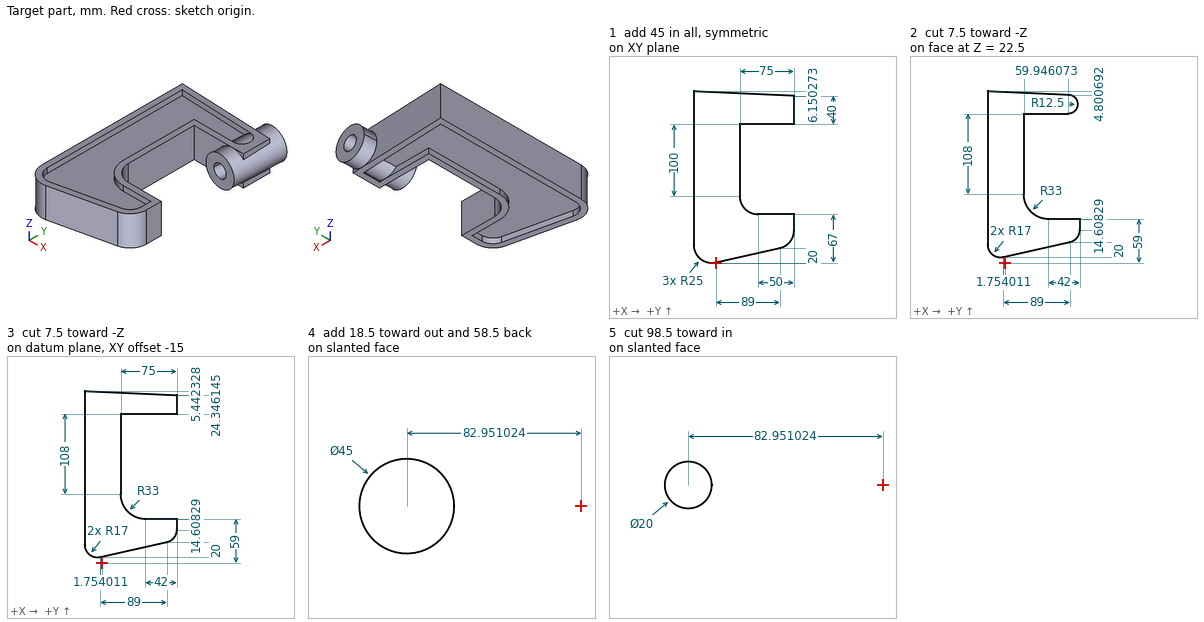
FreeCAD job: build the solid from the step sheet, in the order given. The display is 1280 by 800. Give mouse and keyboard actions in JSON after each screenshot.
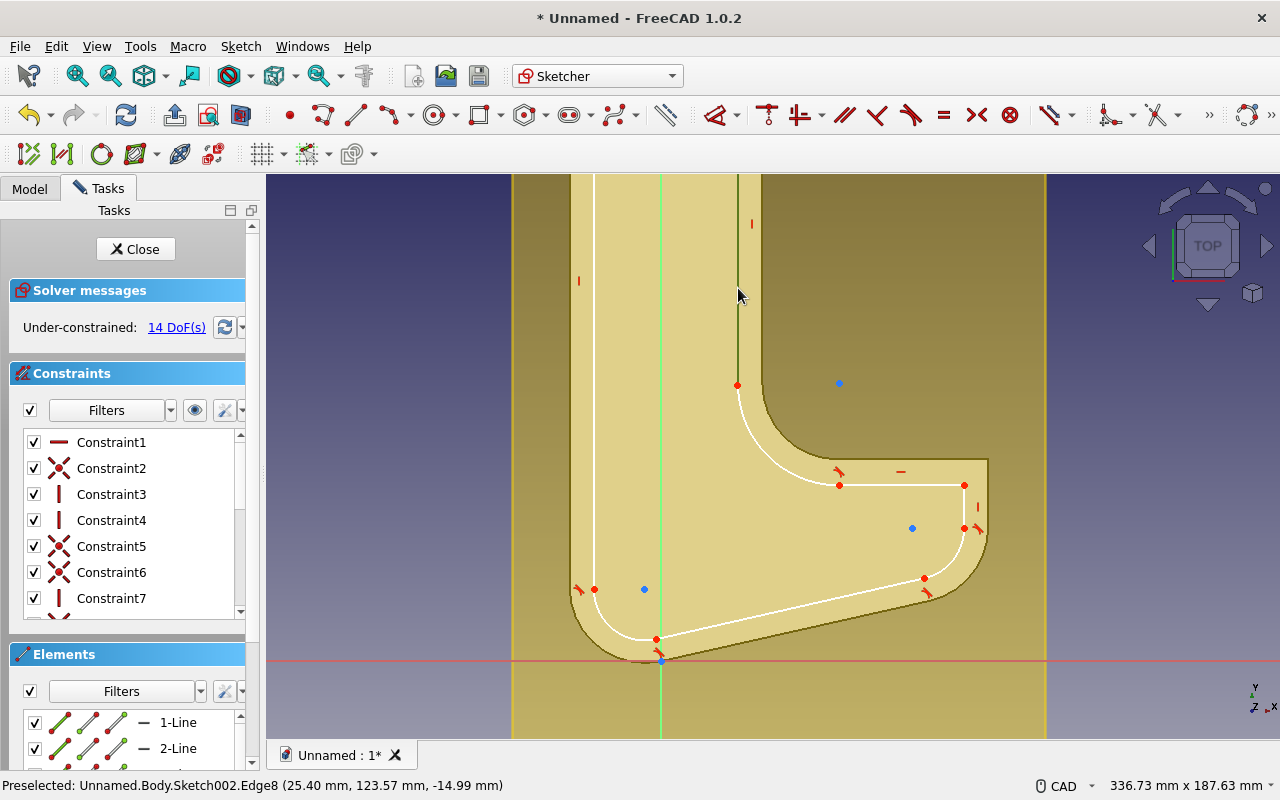
{"action": "left_click", "coordinate": [750, 431]}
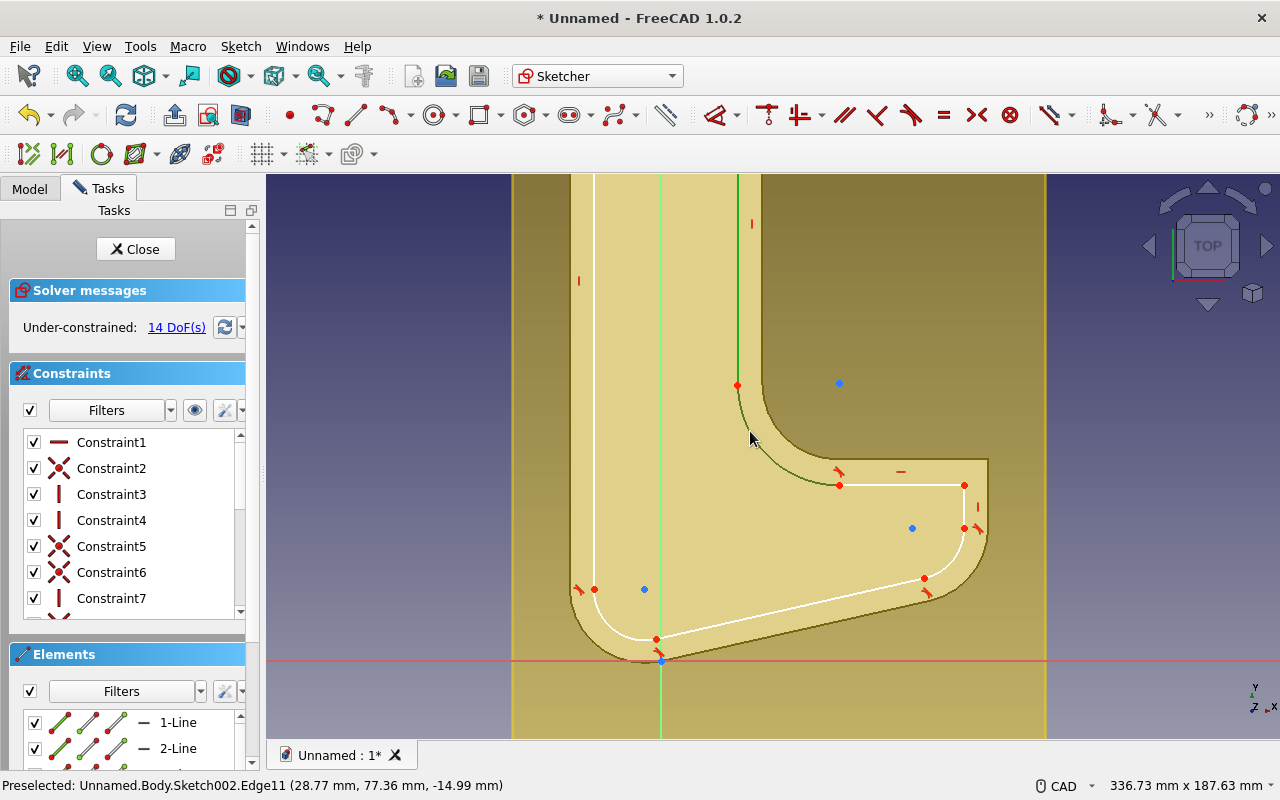
{"action": "left_click", "coordinate": [911, 116]}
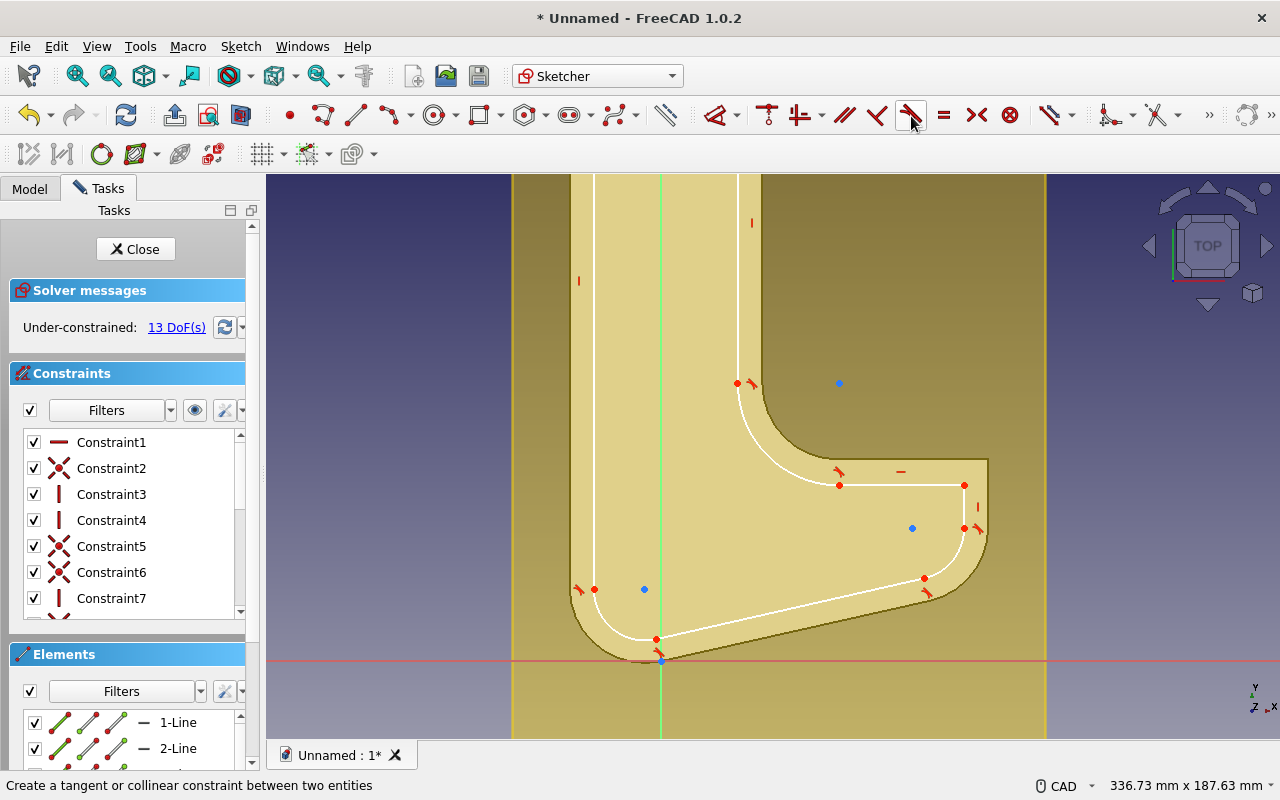
{"action": "left_click", "coordinate": [943, 570]}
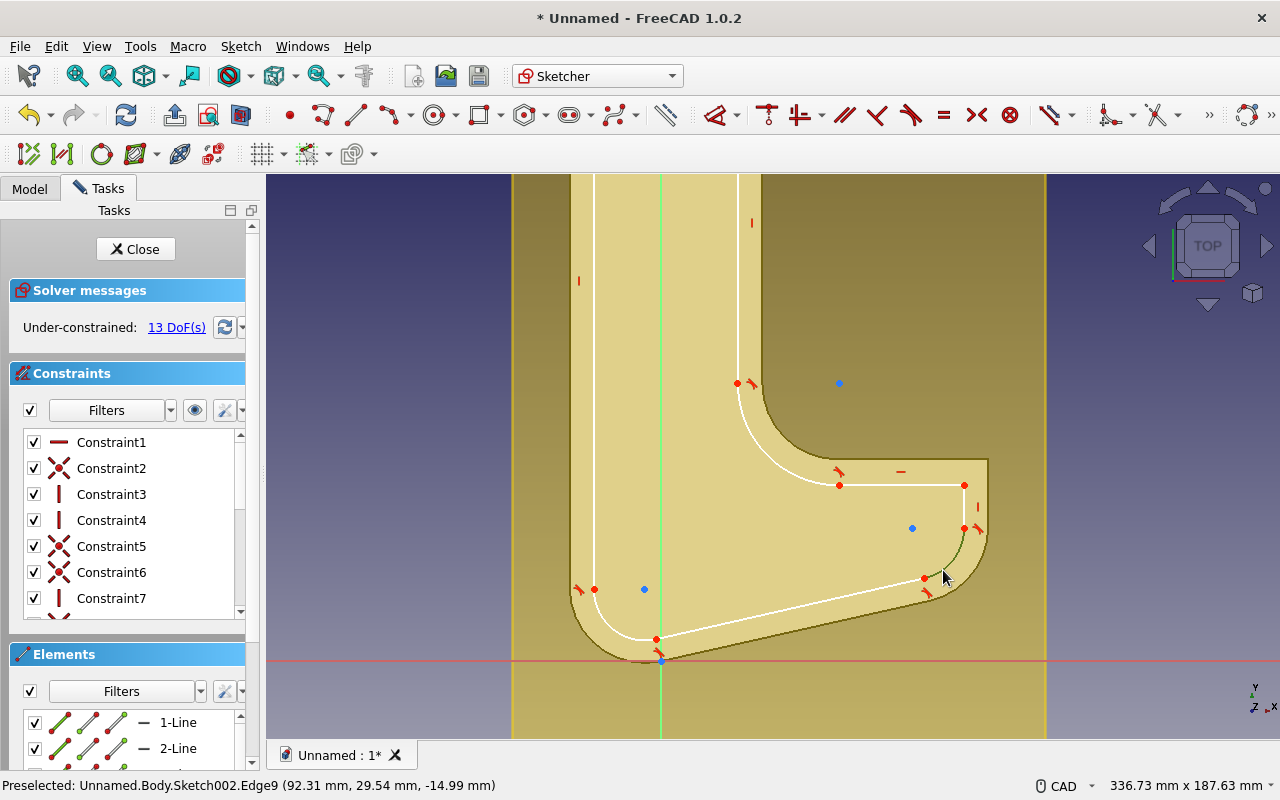
{"action": "left_click", "coordinate": [601, 616]}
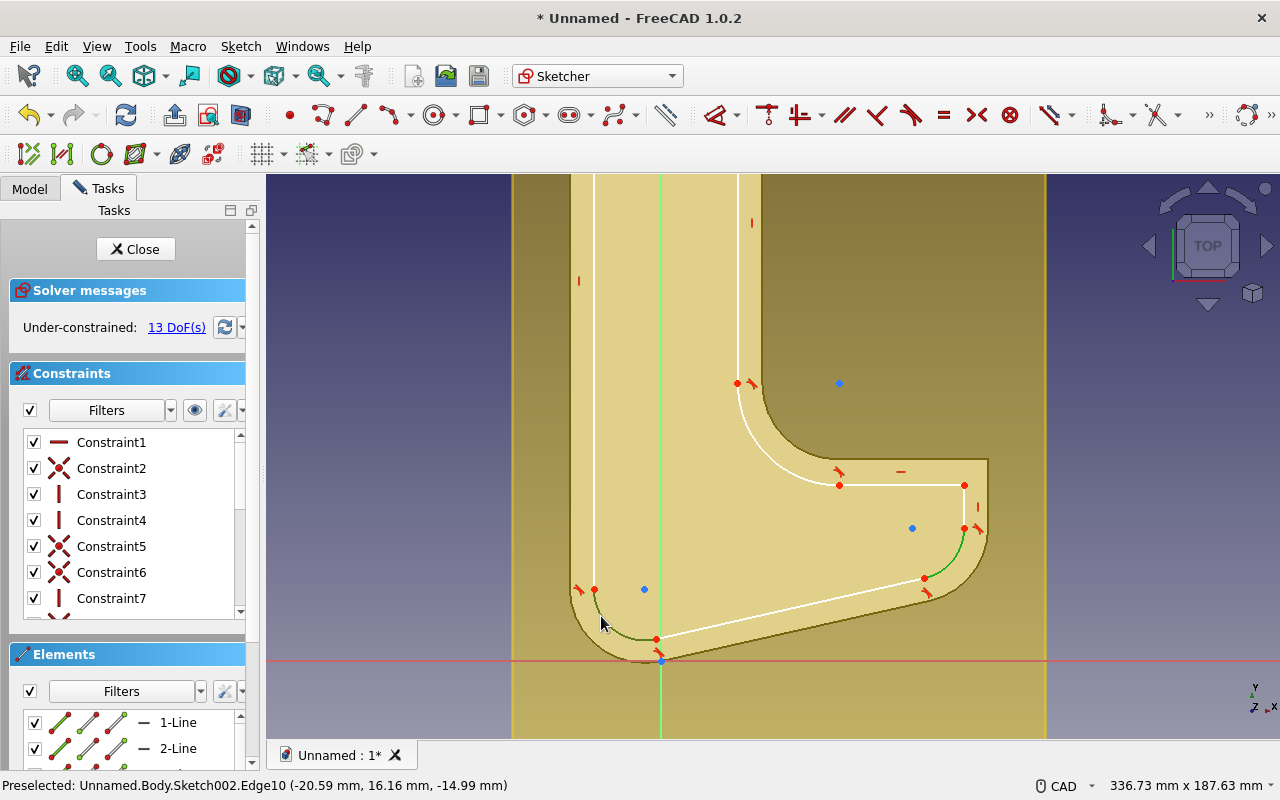
{"action": "left_click", "coordinate": [944, 116]}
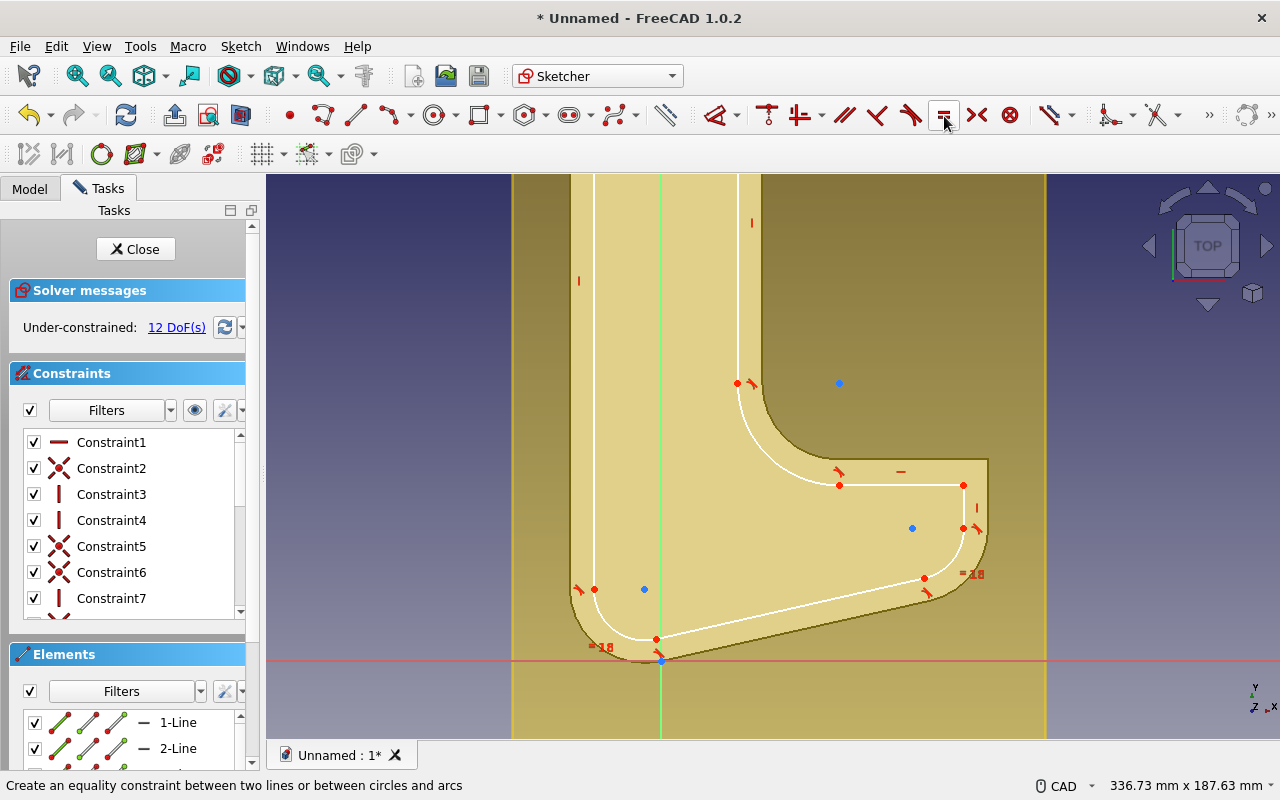
{"action": "left_click", "coordinate": [714, 116]}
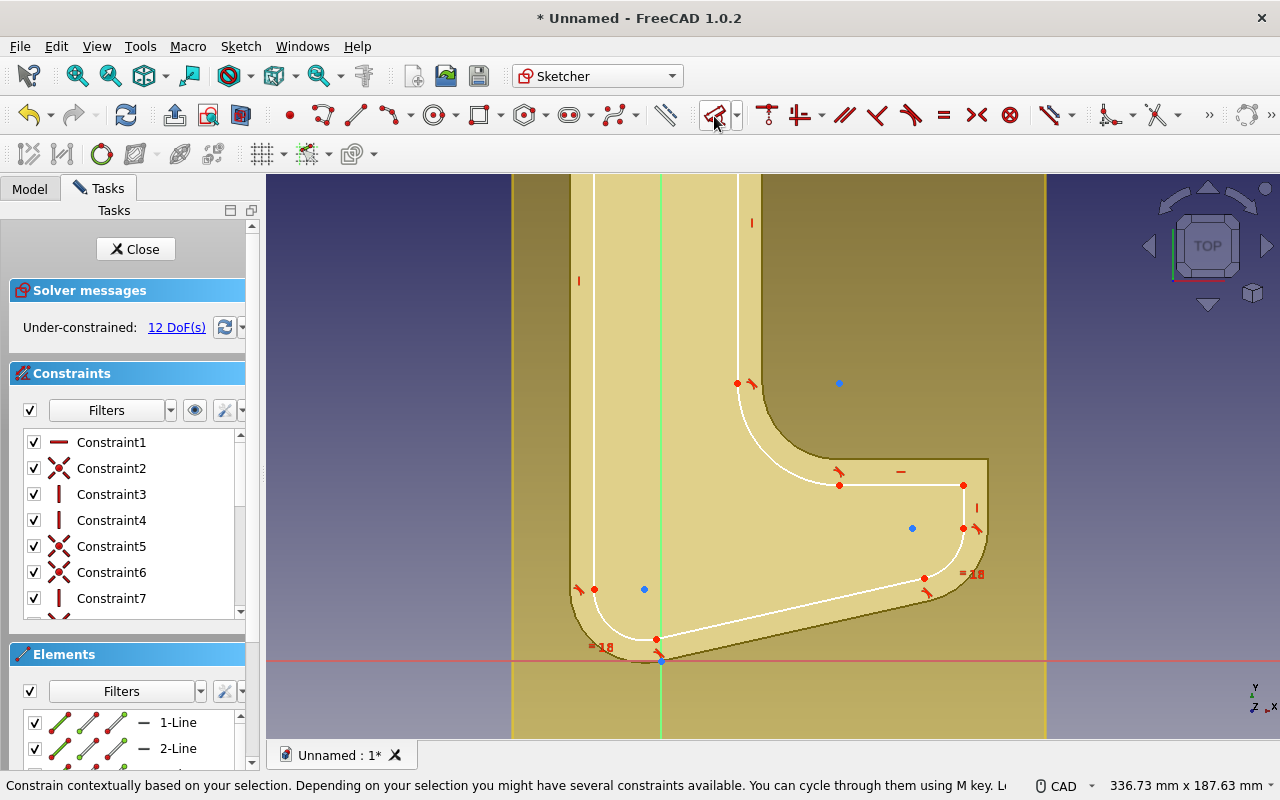
{"action": "left_click", "coordinate": [943, 570]}
{"action": "left_click", "coordinate": [962, 596]}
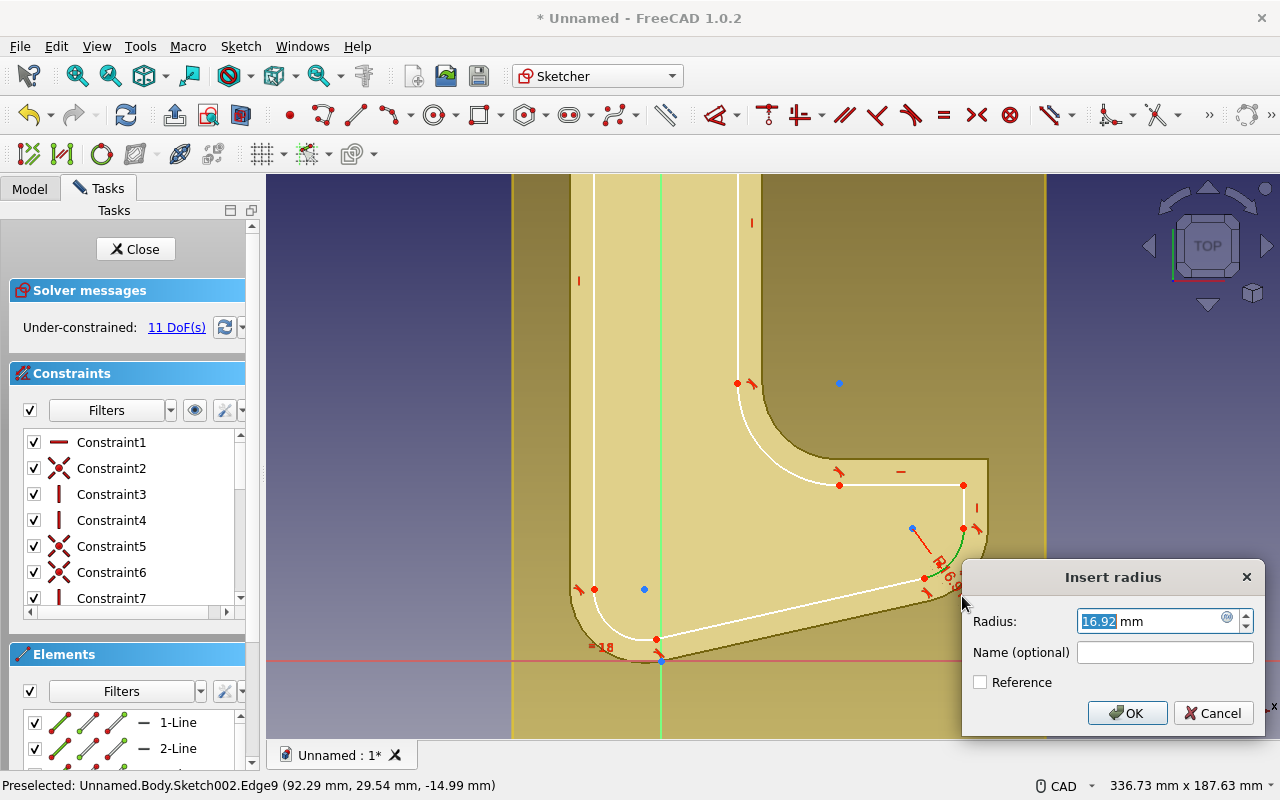
{"action": "type", "text": "17"}
{"action": "key", "text": "Return"}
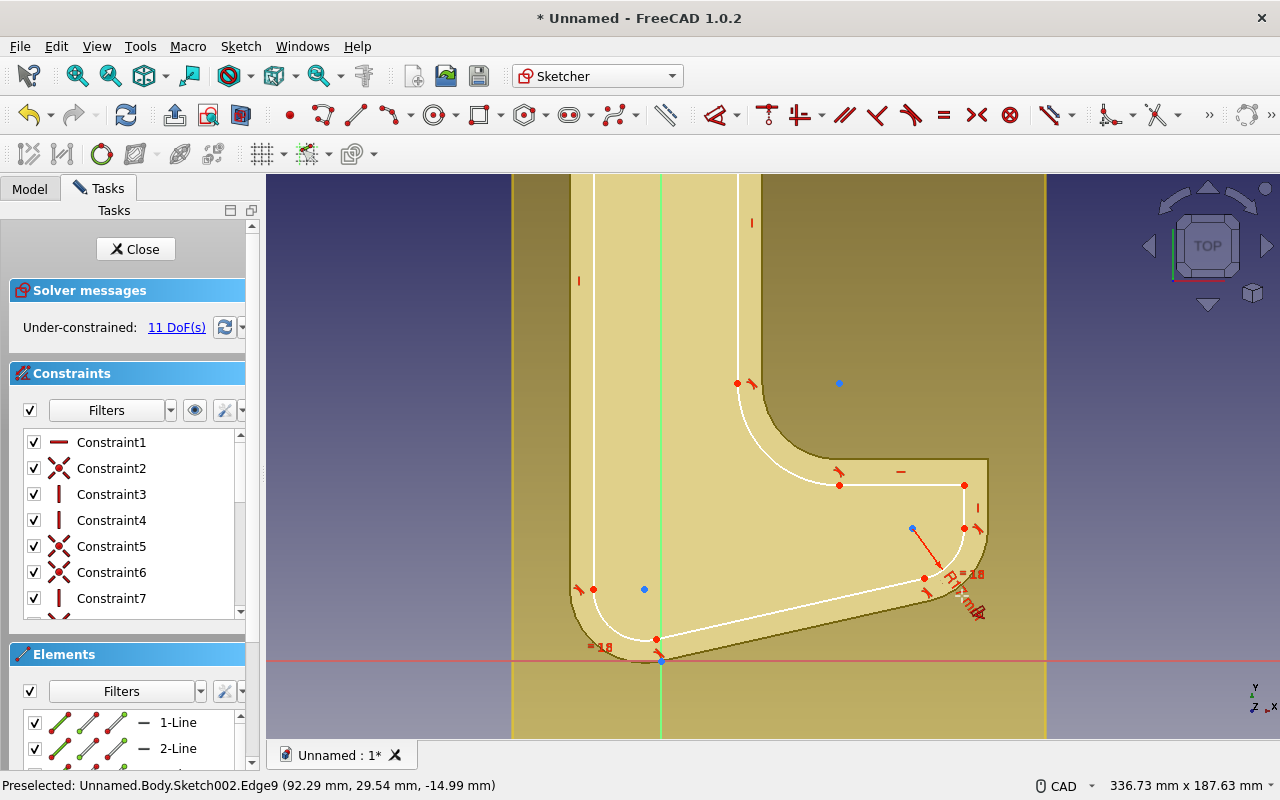
{"action": "left_click", "coordinate": [749, 430]}
{"action": "left_click", "coordinate": [720, 445]}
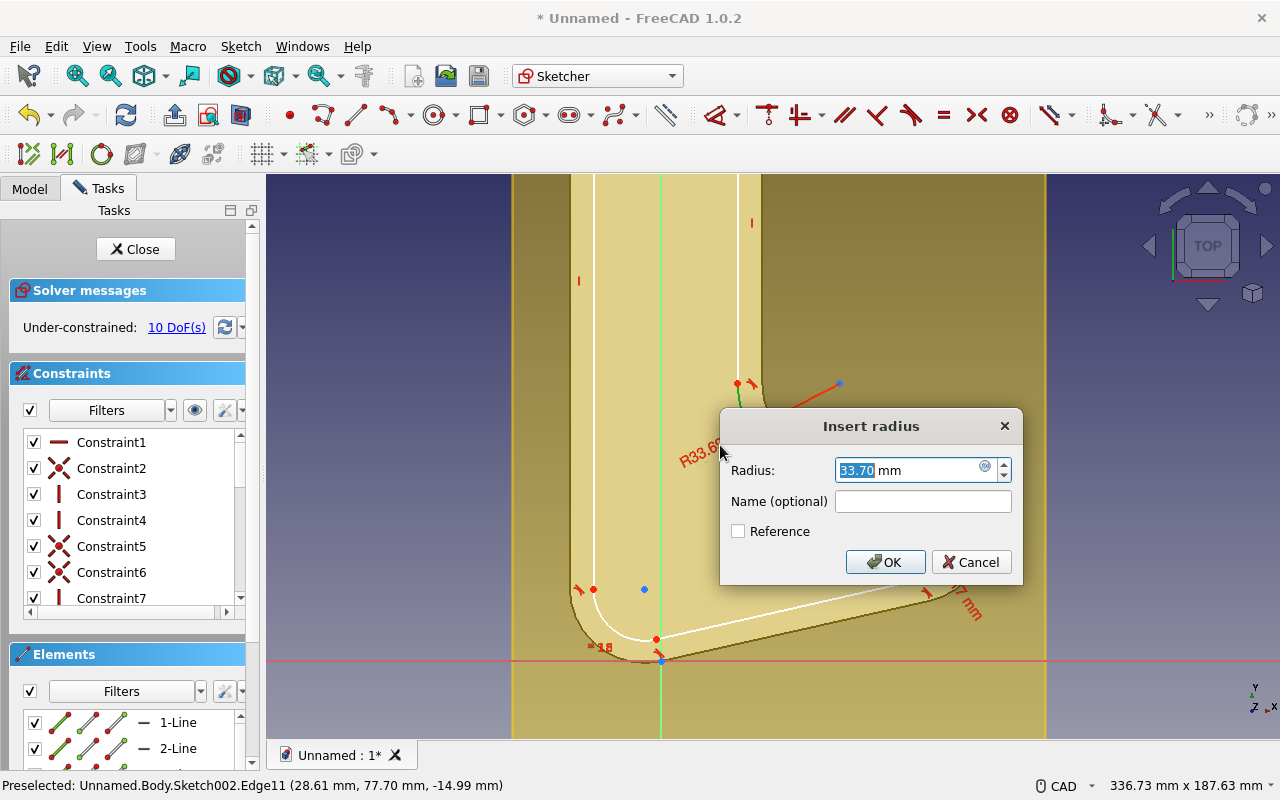
{"action": "type", "text": "33"}
{"action": "key", "text": "Return"}